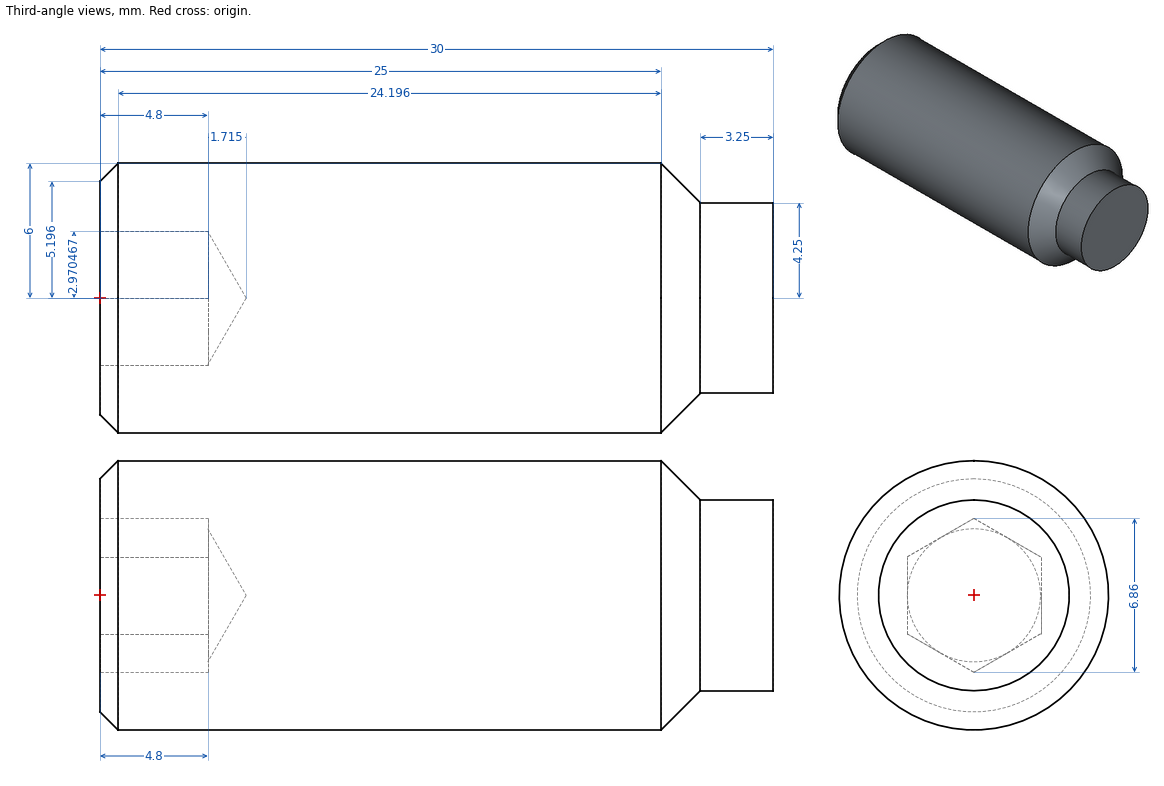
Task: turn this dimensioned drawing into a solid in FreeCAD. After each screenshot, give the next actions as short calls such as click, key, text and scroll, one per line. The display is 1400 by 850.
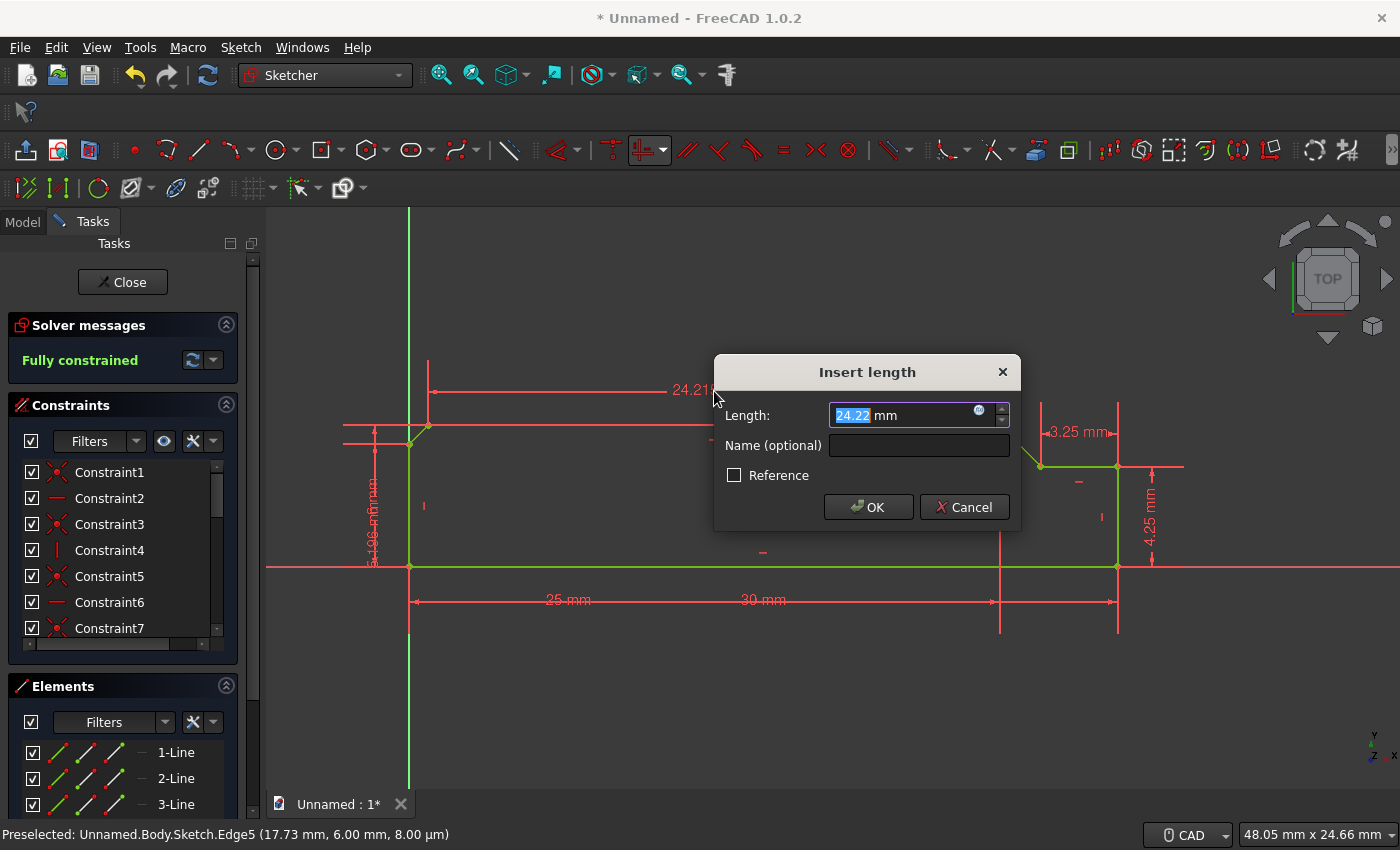
text(24.196)
key(Return)
key(Escape)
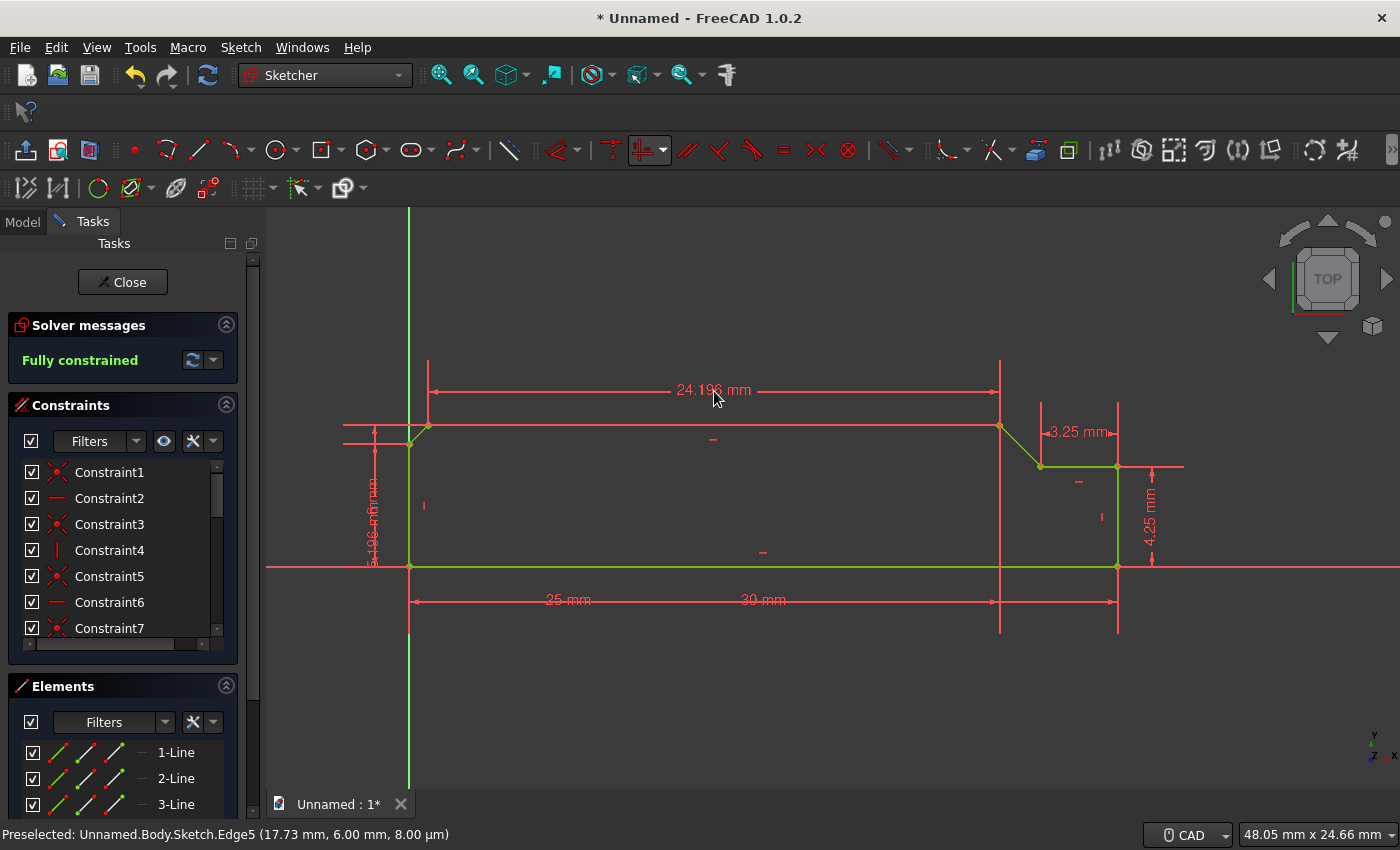
click(123, 282)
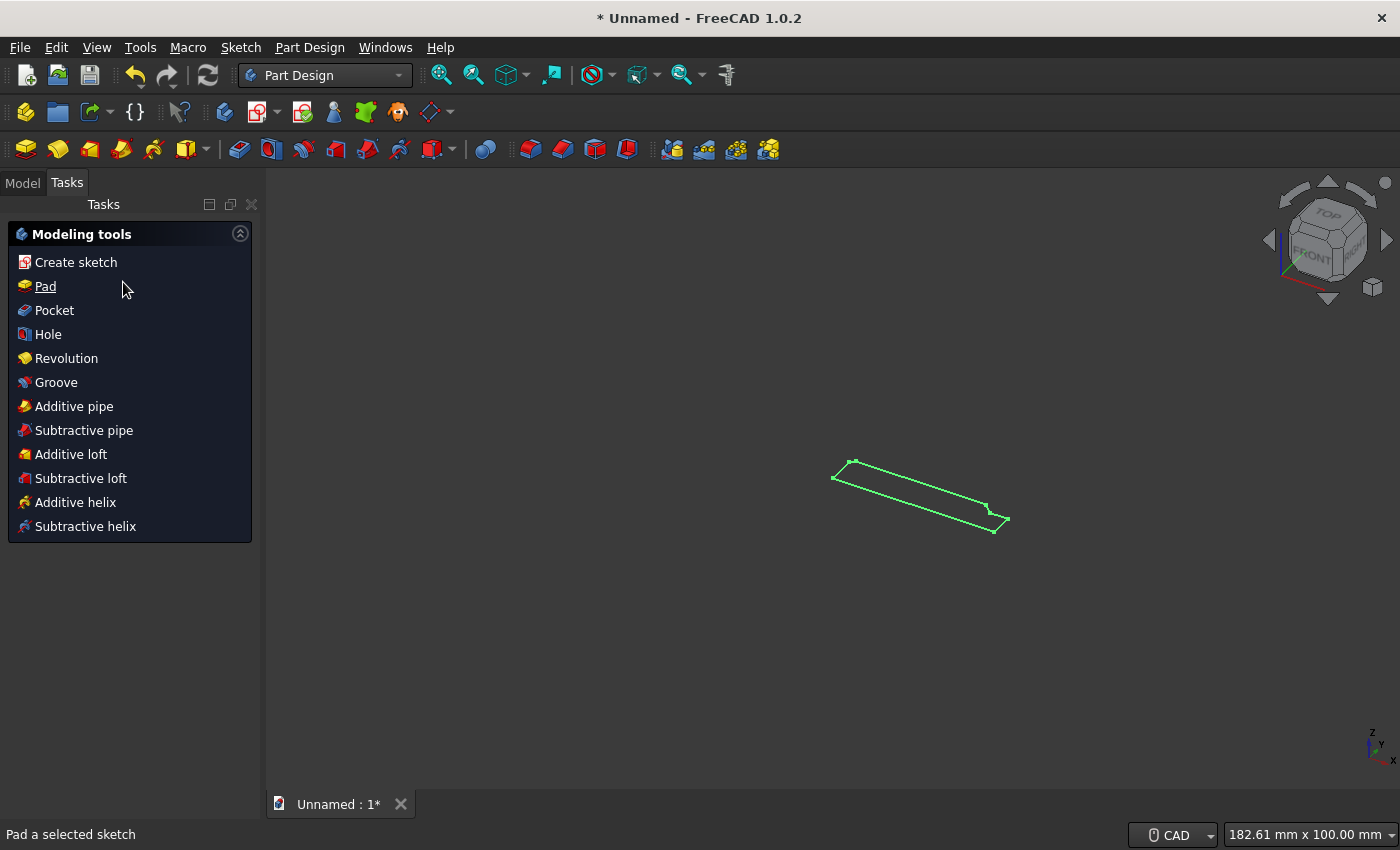
click(58, 150)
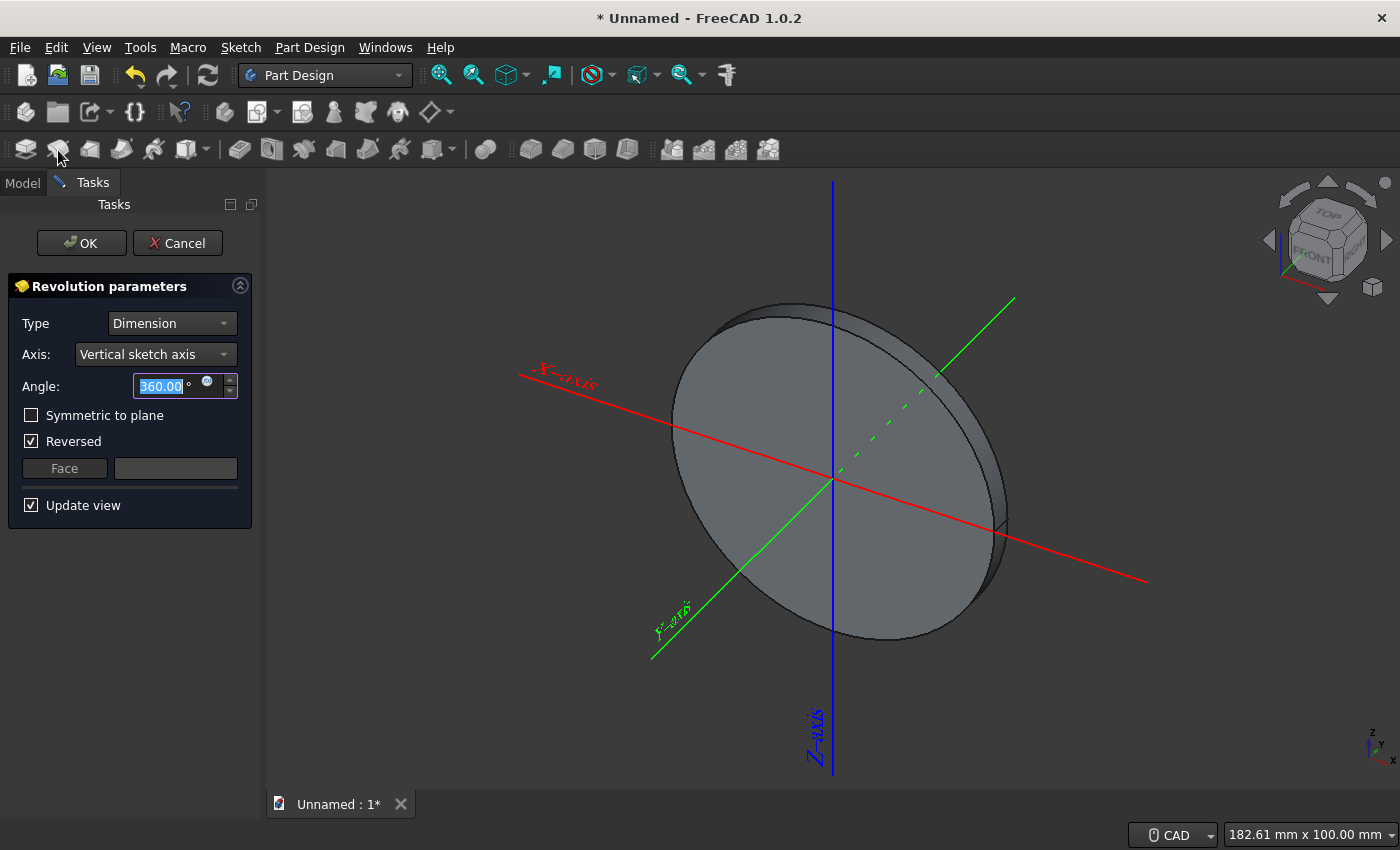
click(156, 354)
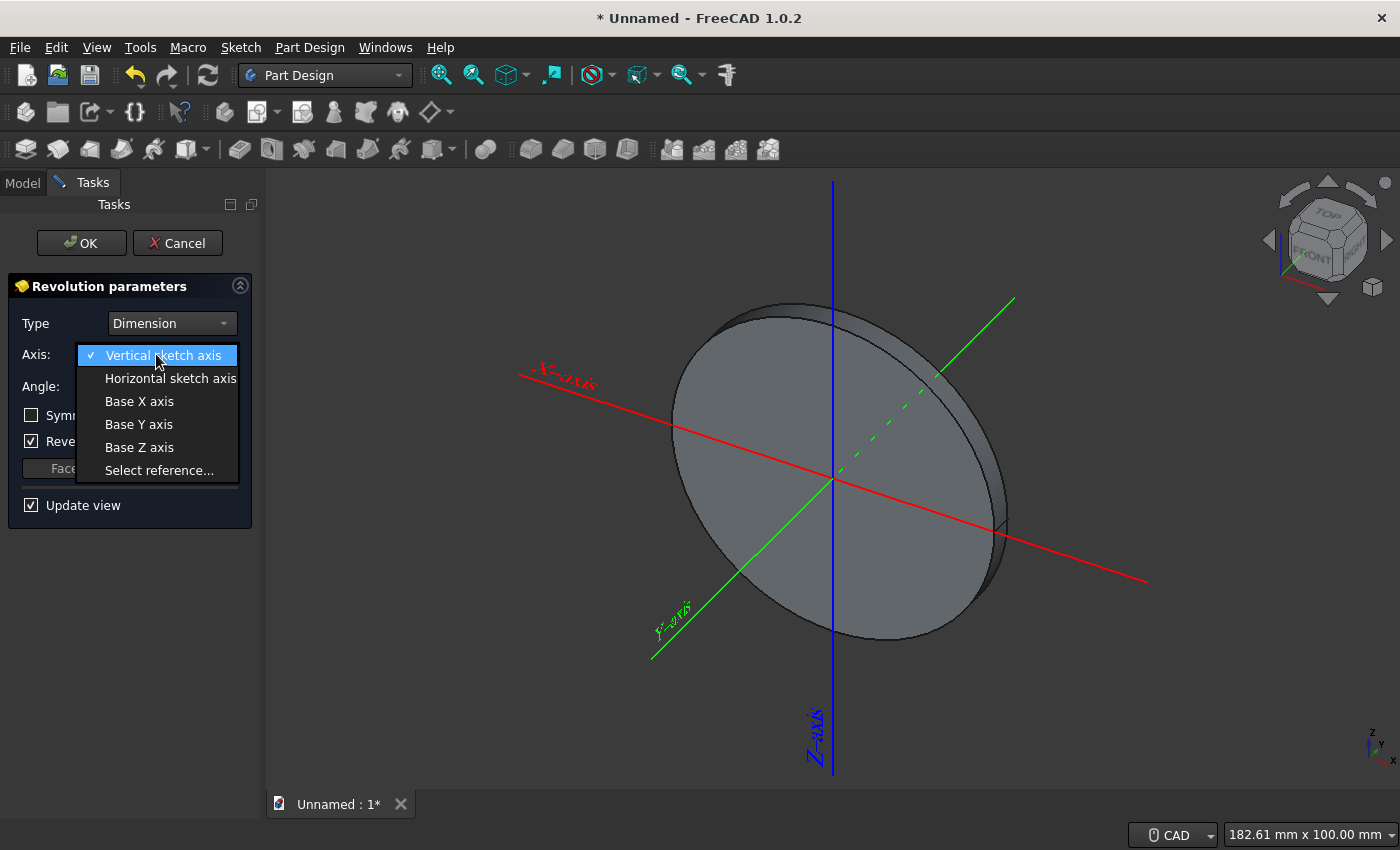
click(156, 378)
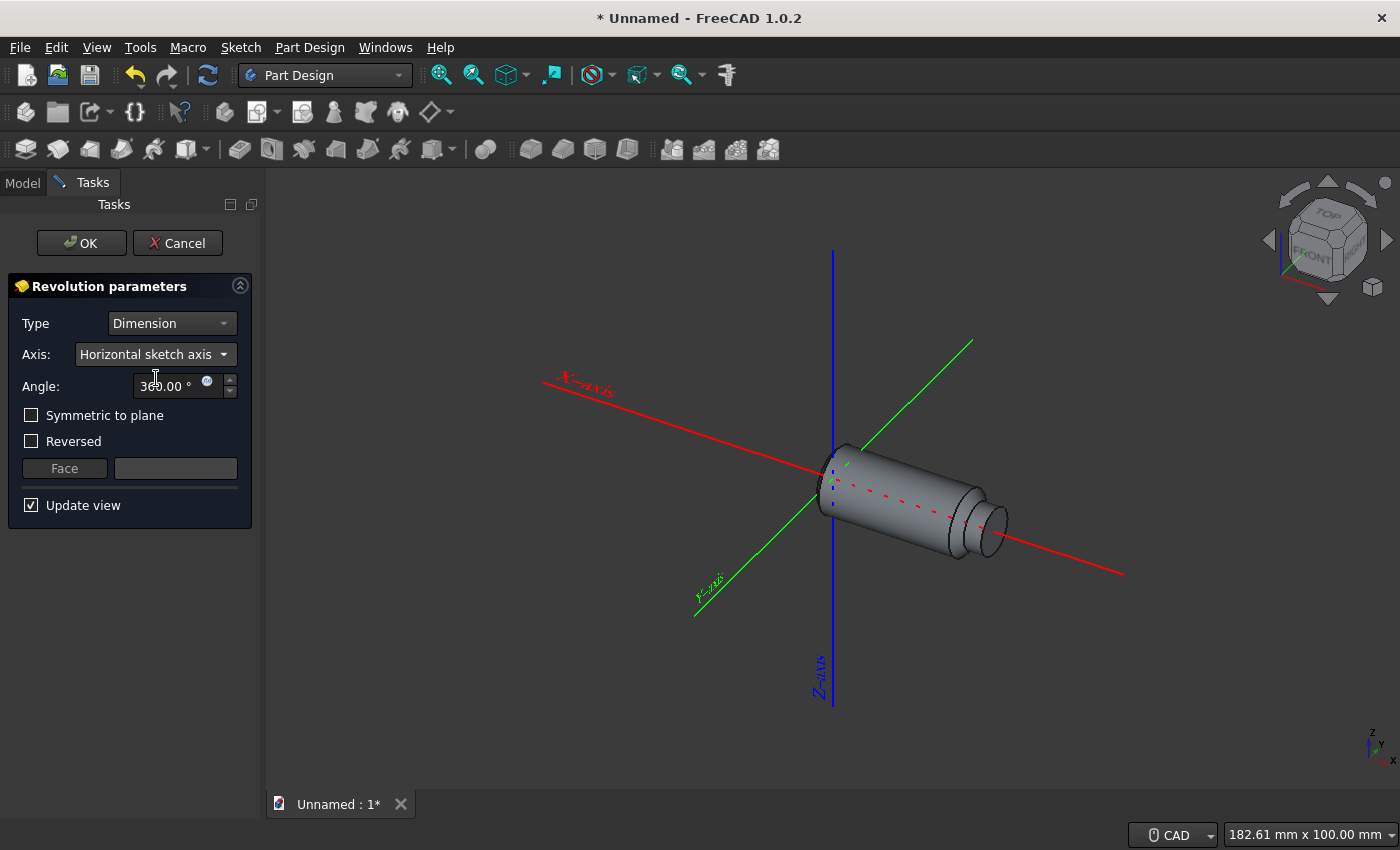
click(82, 243)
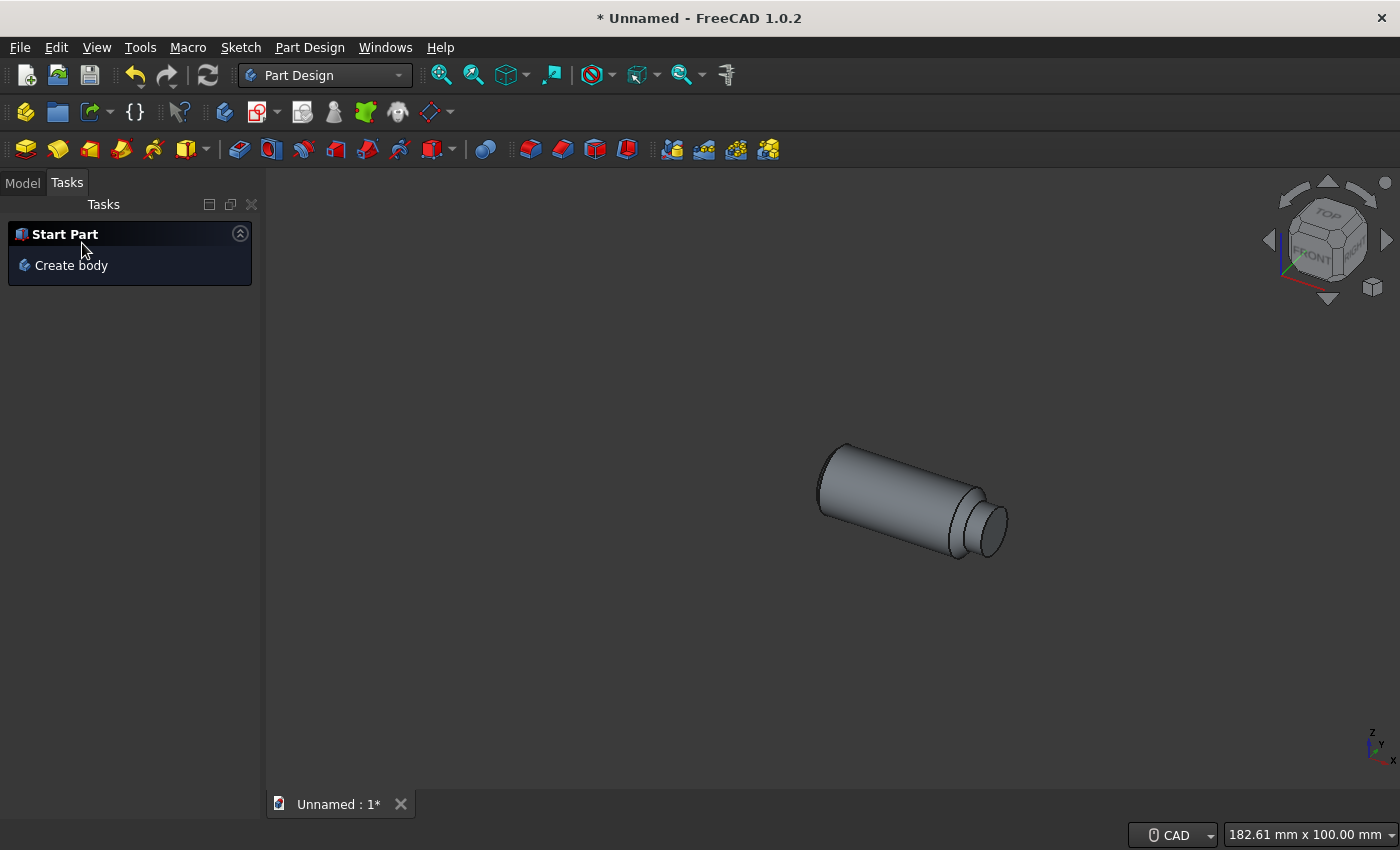
click(442, 76)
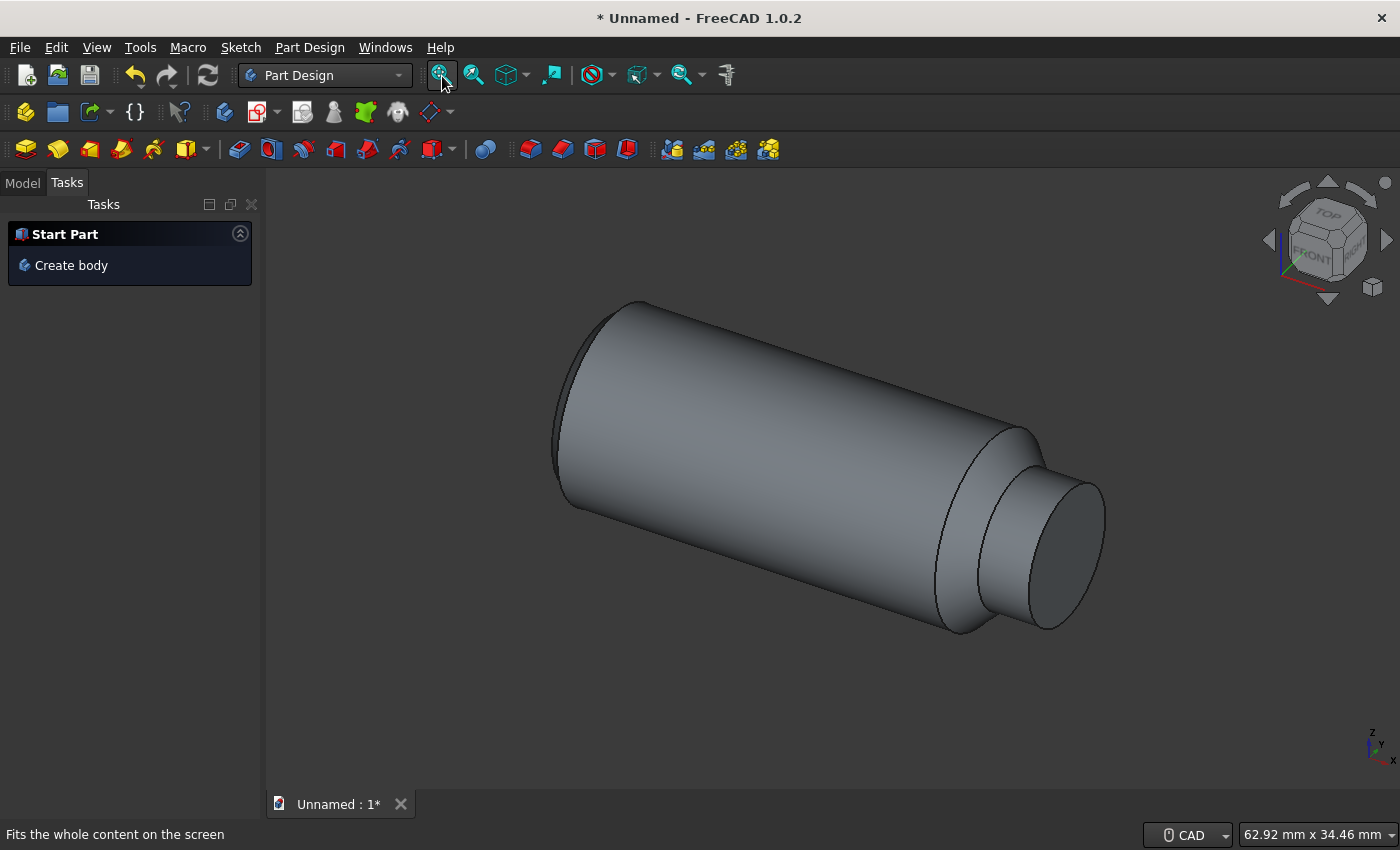
click(258, 112)